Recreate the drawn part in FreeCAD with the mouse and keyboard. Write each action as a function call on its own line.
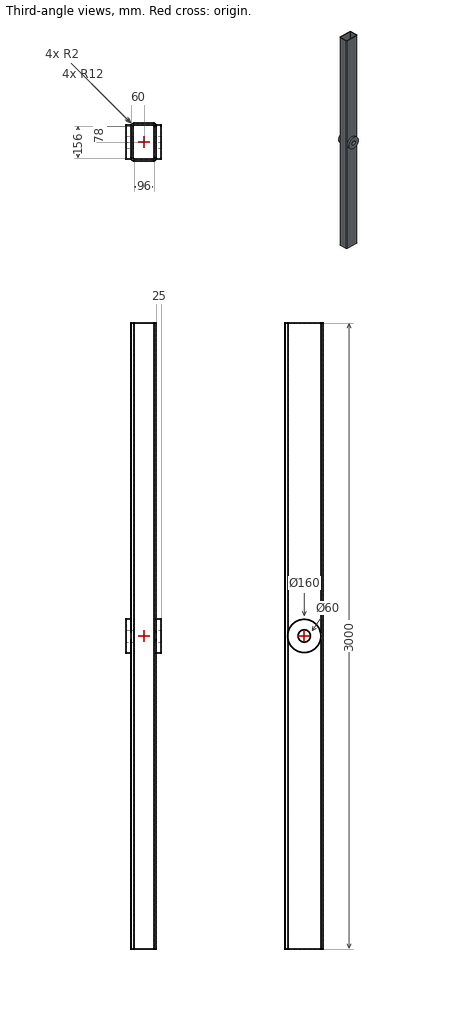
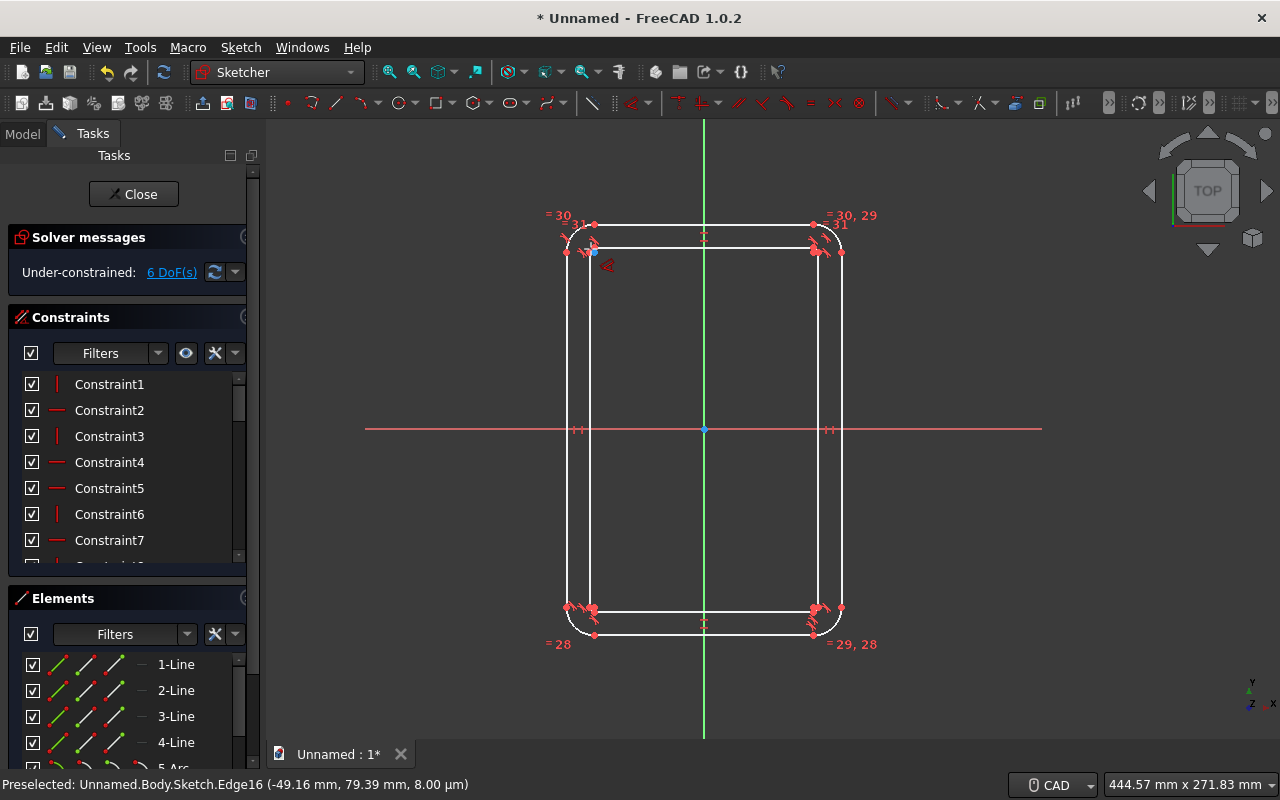
scroll(570, 620, up, 2)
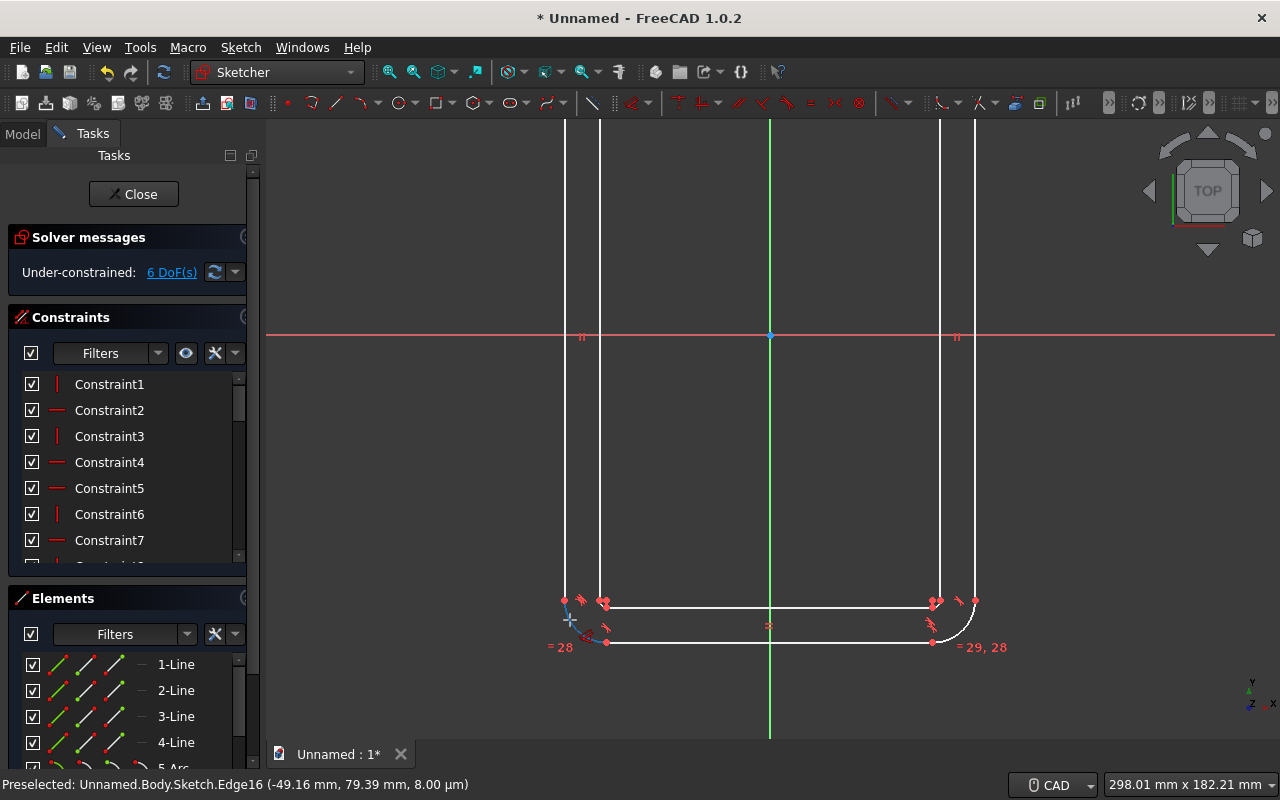
click(569, 620)
click(541, 635)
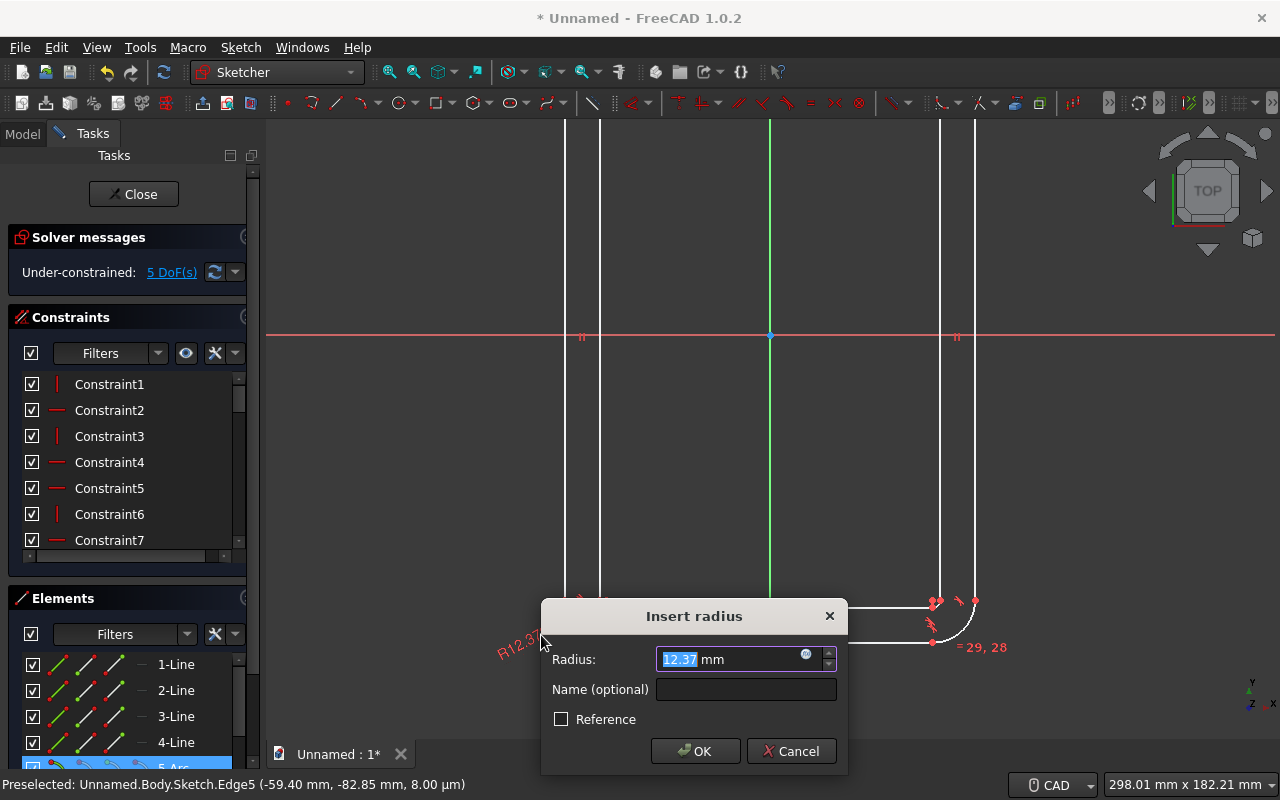
text(12)
key(Return)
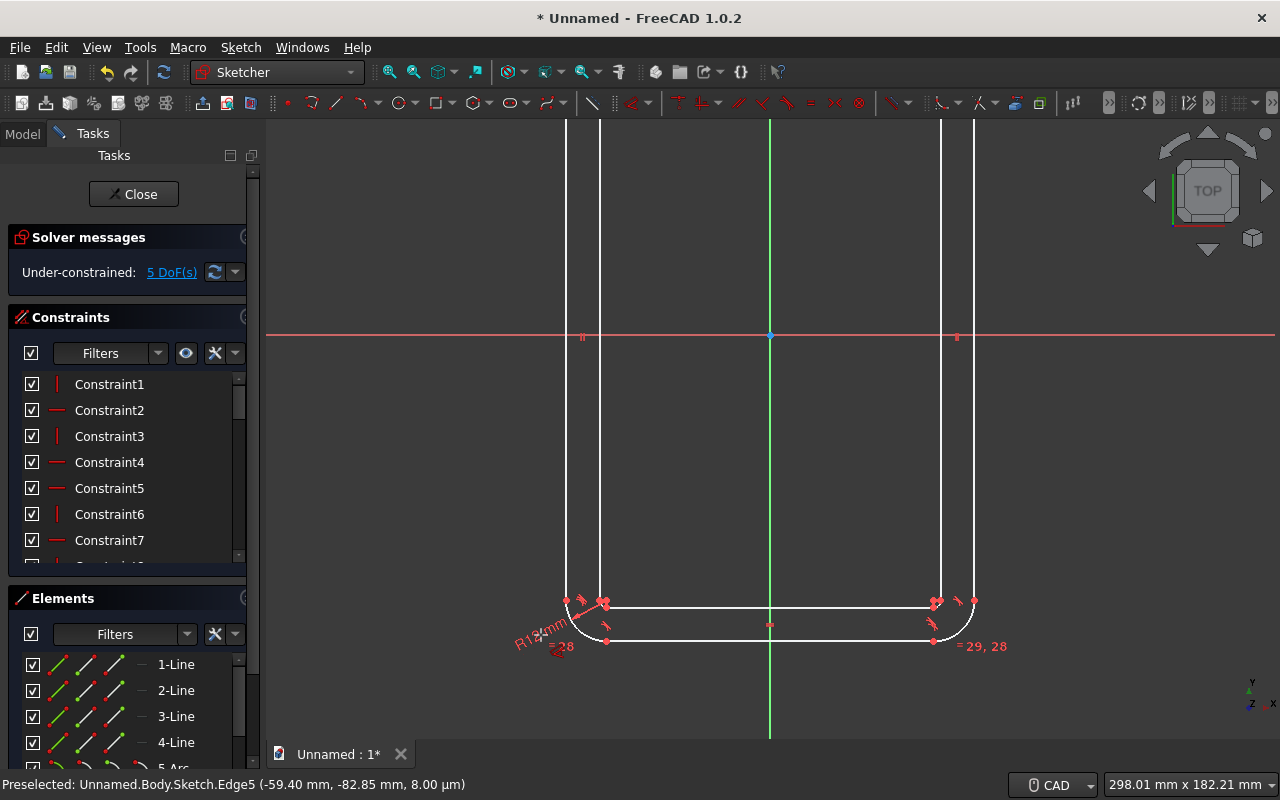
scroll(571, 619, down, 2)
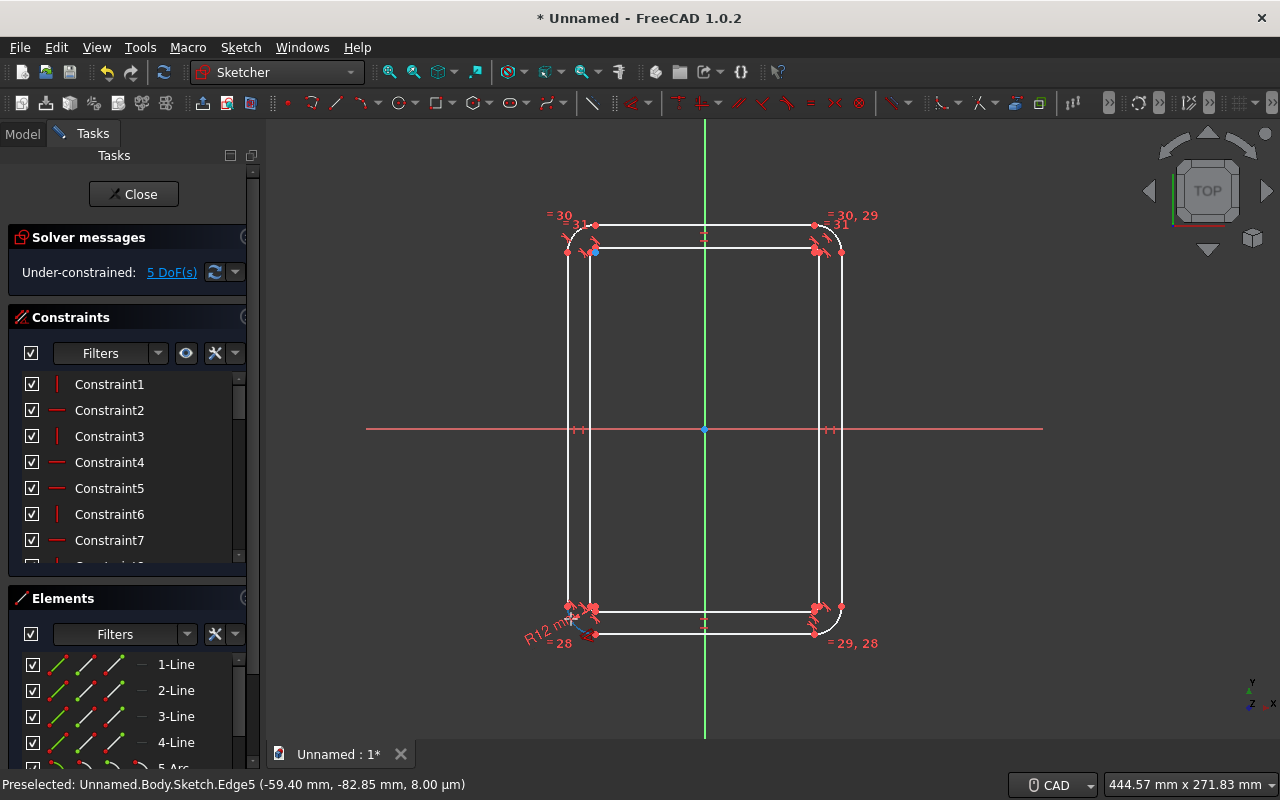
scroll(818, 249, up, 11)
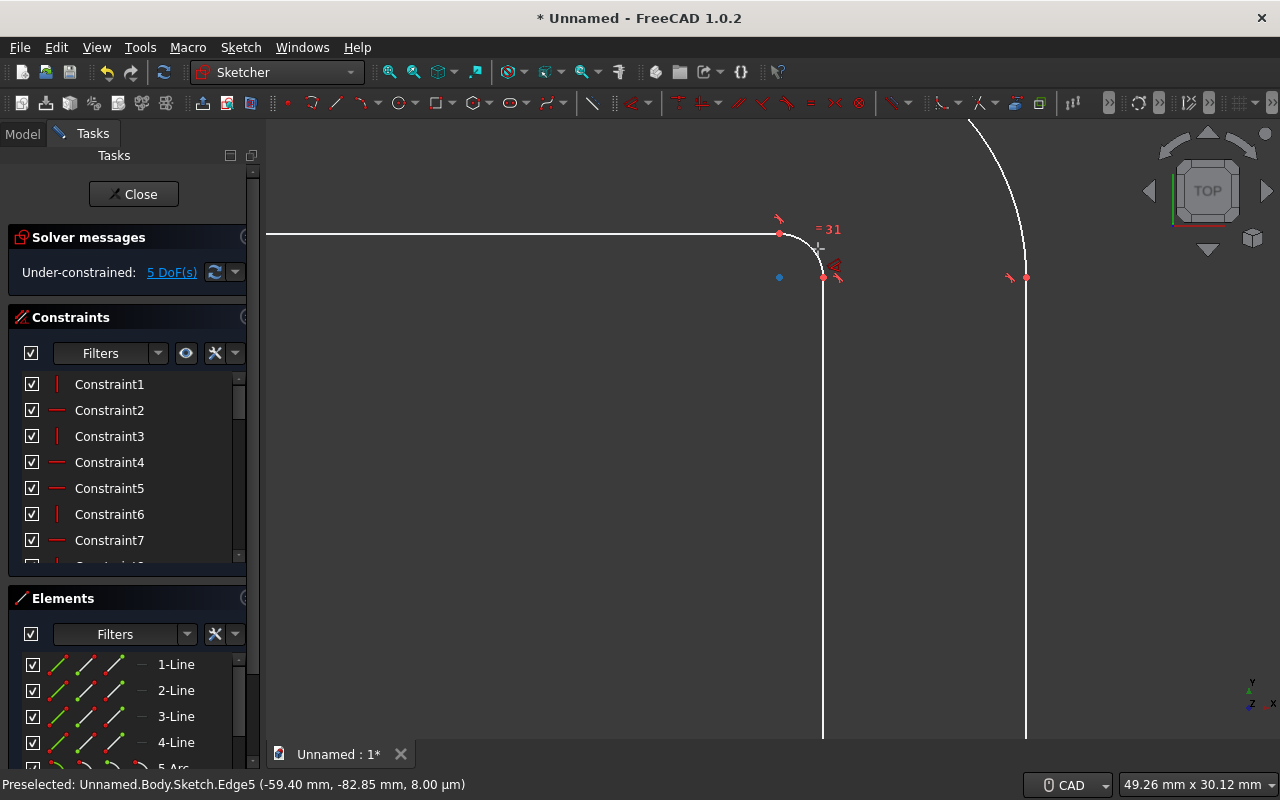
click(810, 247)
click(833, 224)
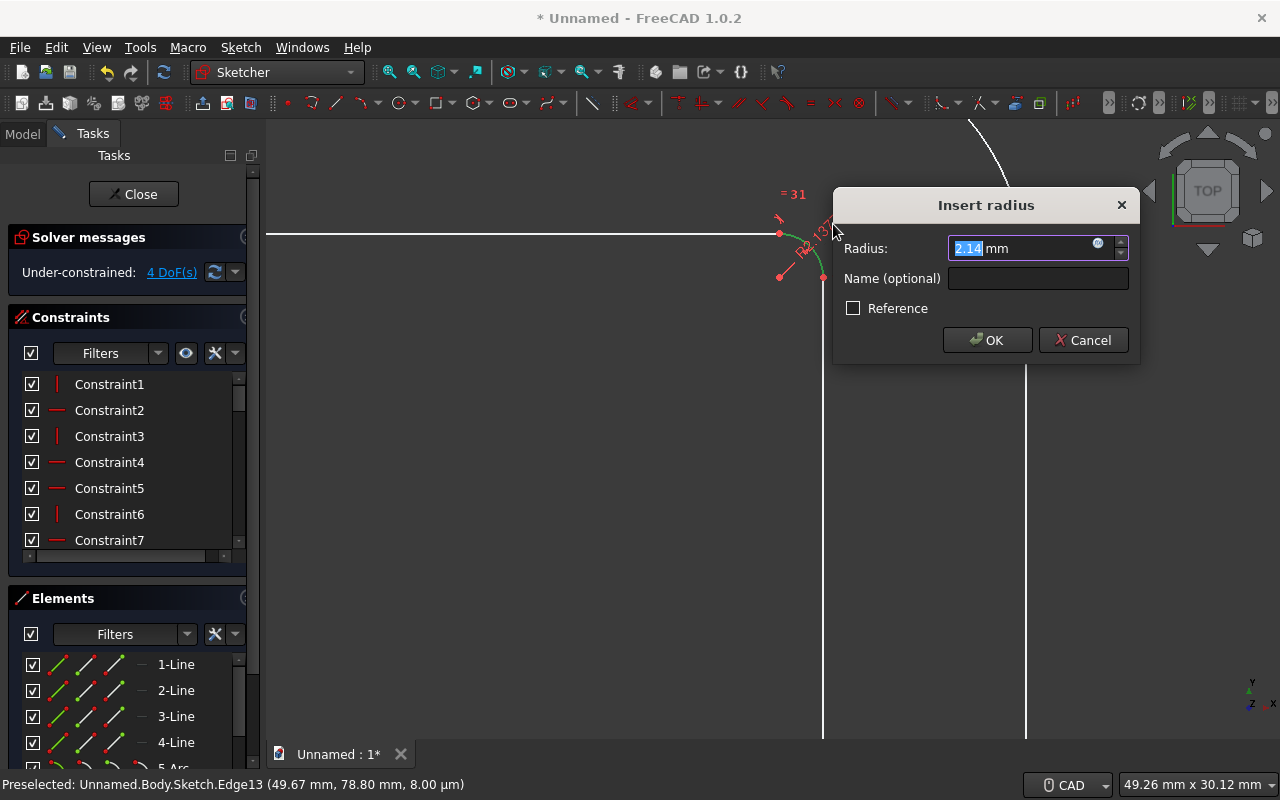
text(2)
key(Return)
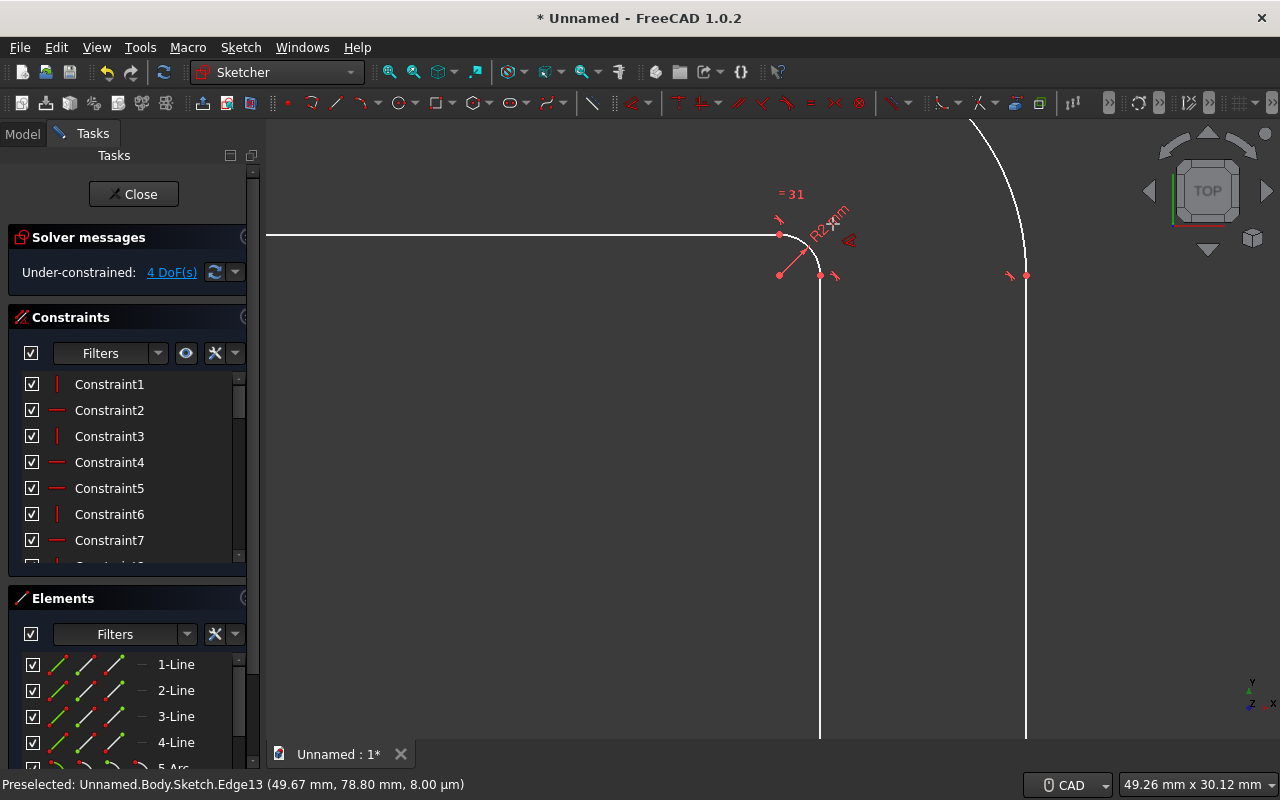
scroll(818, 249, down, 11)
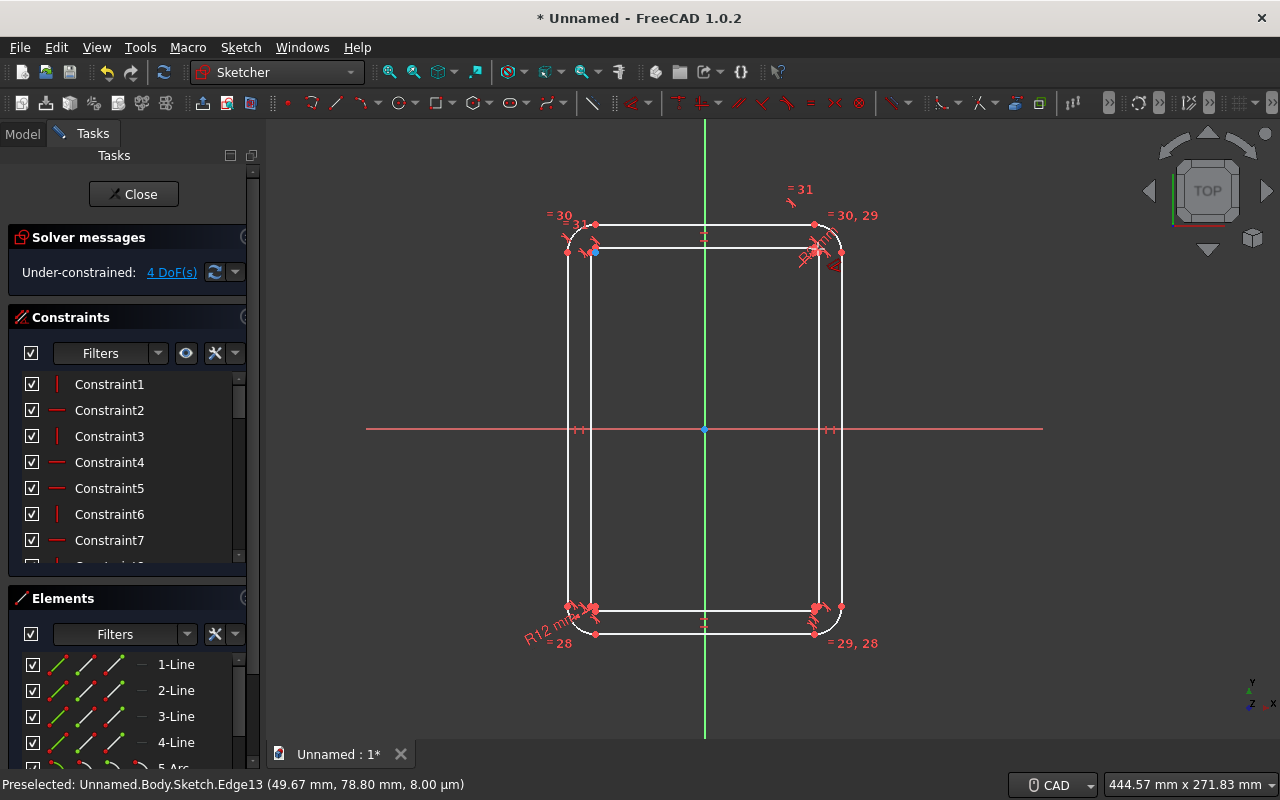
click(661, 634)
click(654, 668)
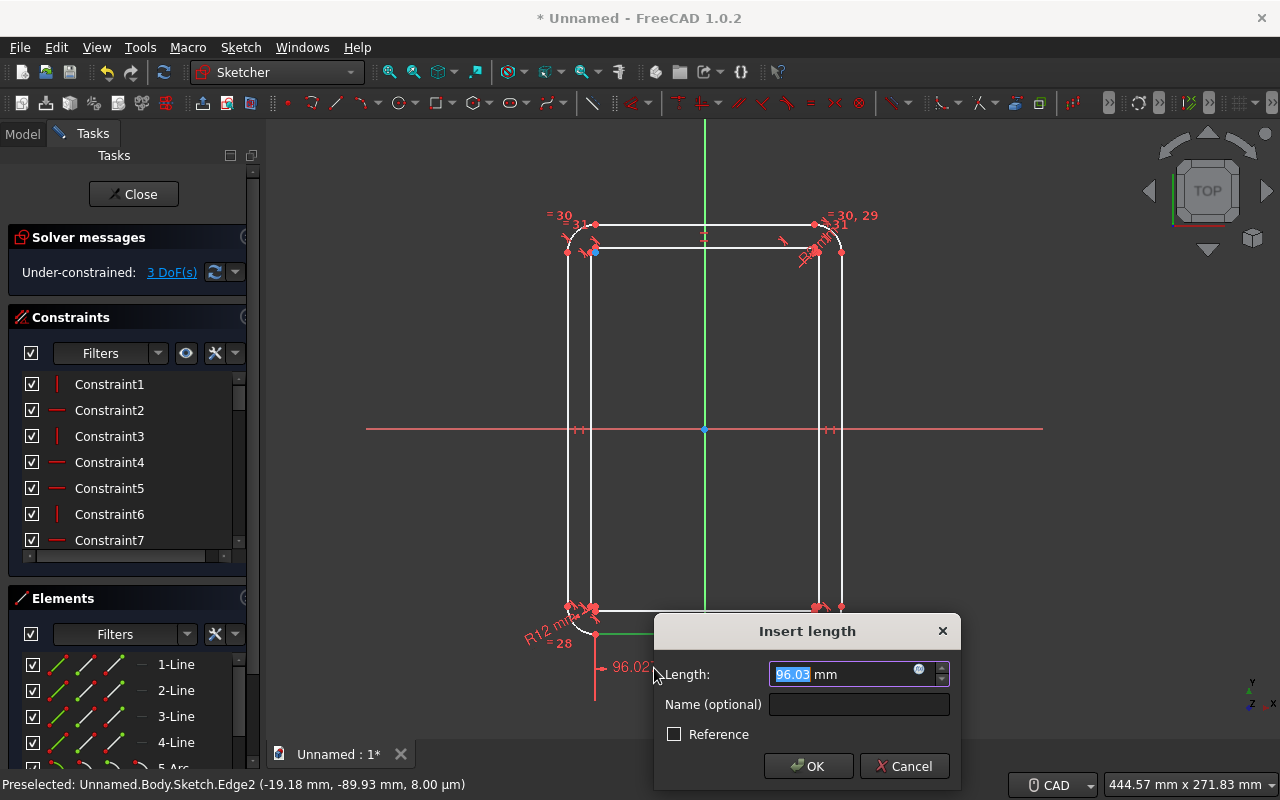
text(96)
key(Return)